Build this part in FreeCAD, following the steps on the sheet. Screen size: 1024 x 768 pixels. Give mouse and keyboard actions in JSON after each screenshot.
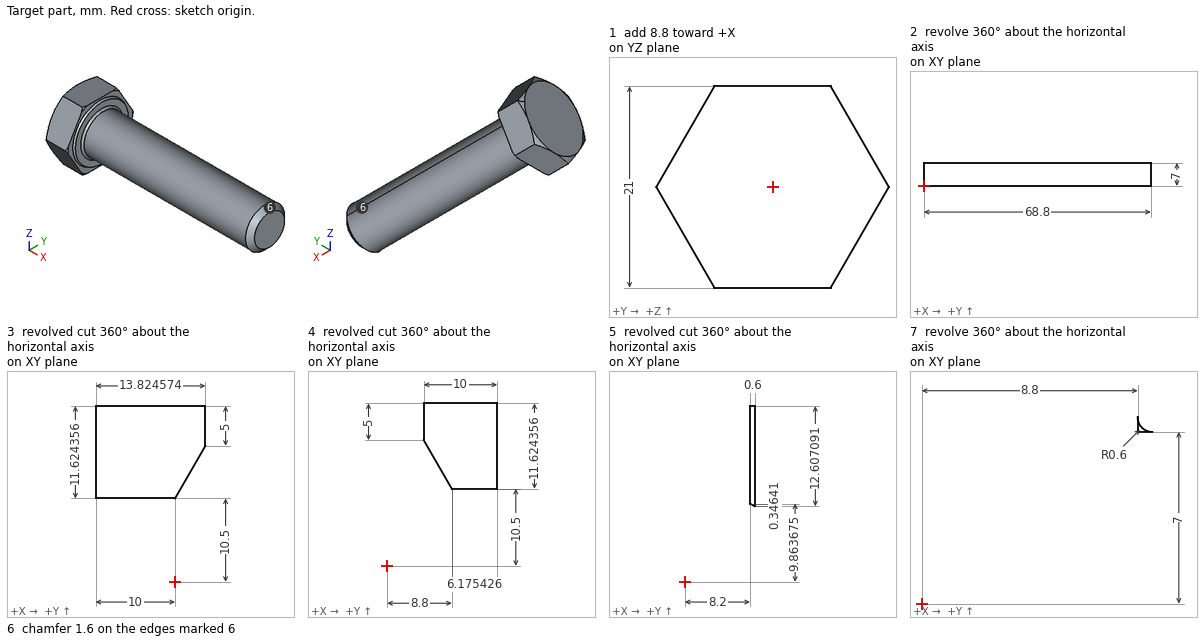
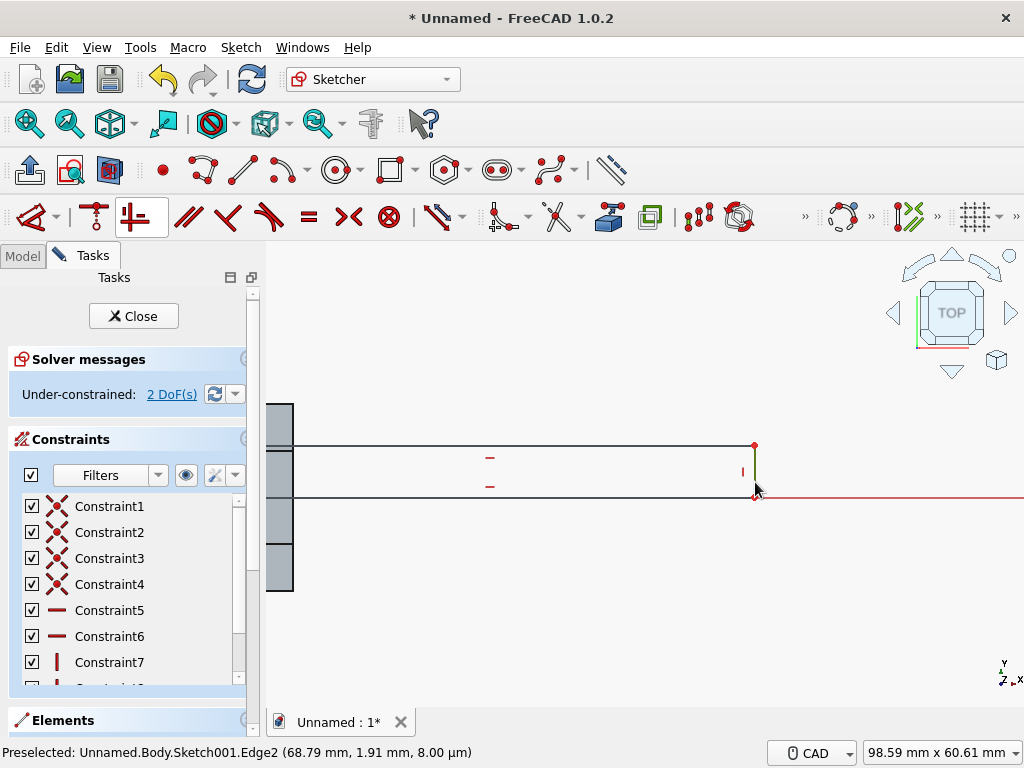
{"action": "left_click", "coordinate": [58, 218]}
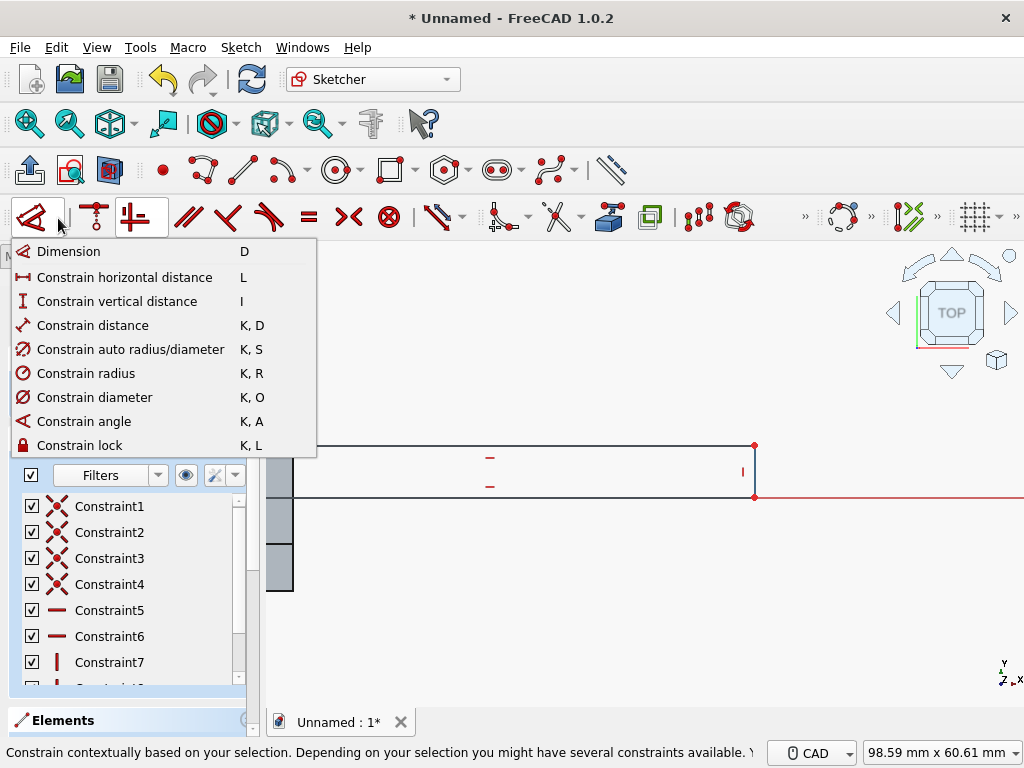
{"action": "left_click", "coordinate": [164, 301]}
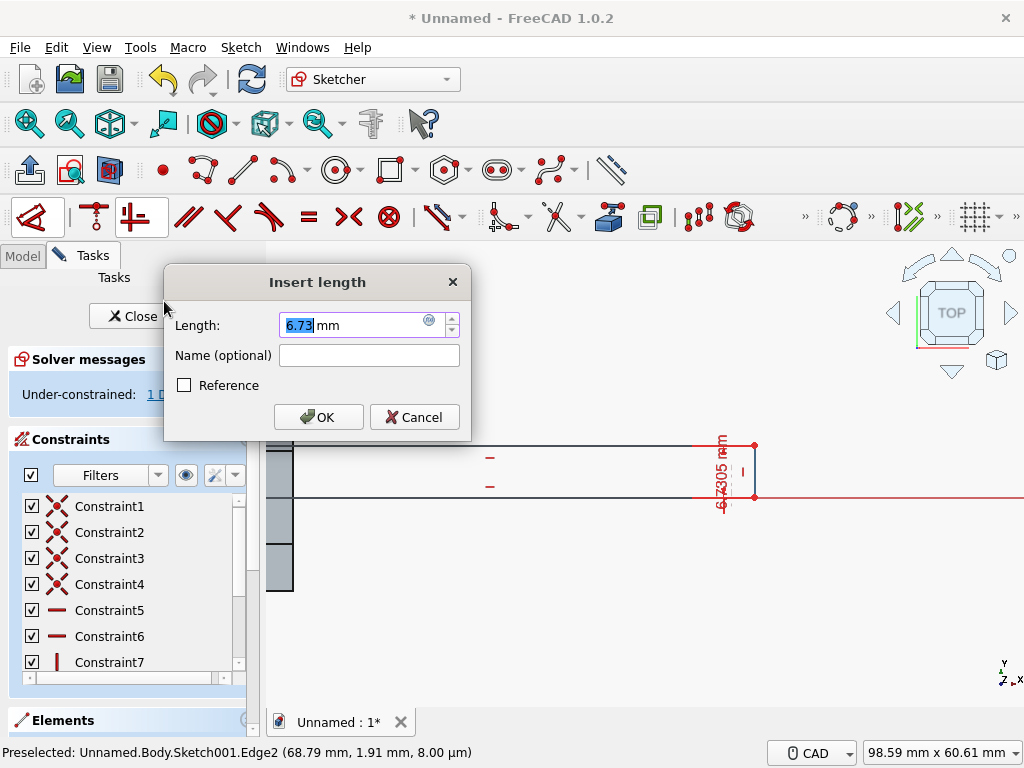
{"action": "type", "text": "7"}
{"action": "key", "text": "Return"}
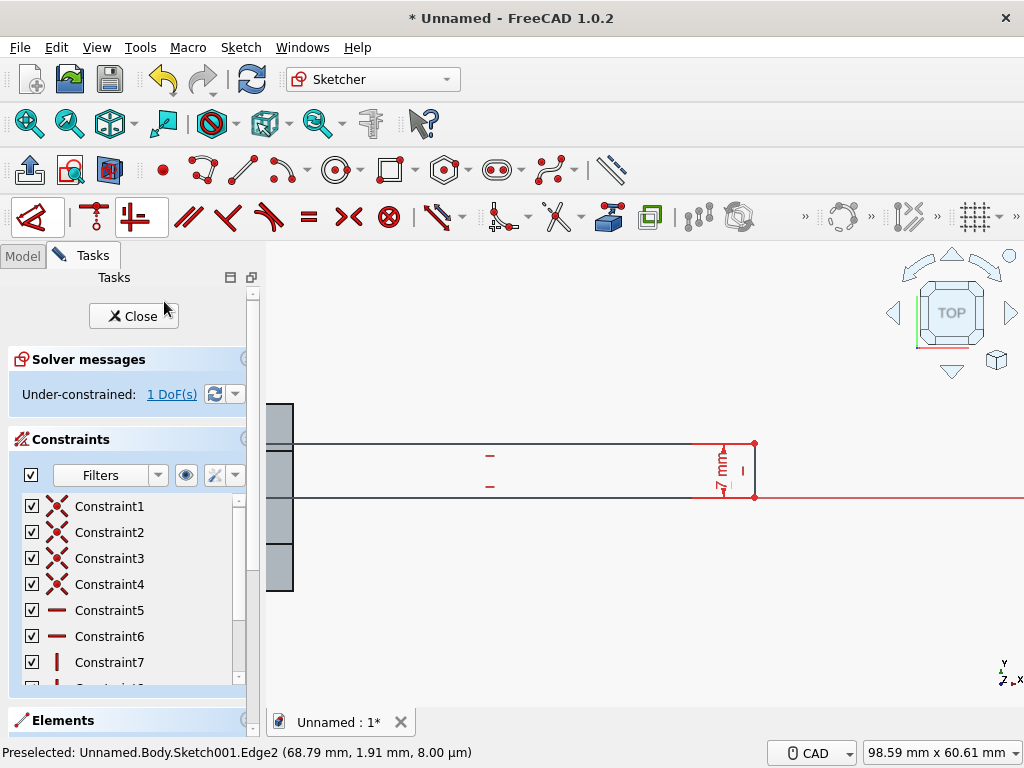
{"action": "left_click", "coordinate": [384, 498]}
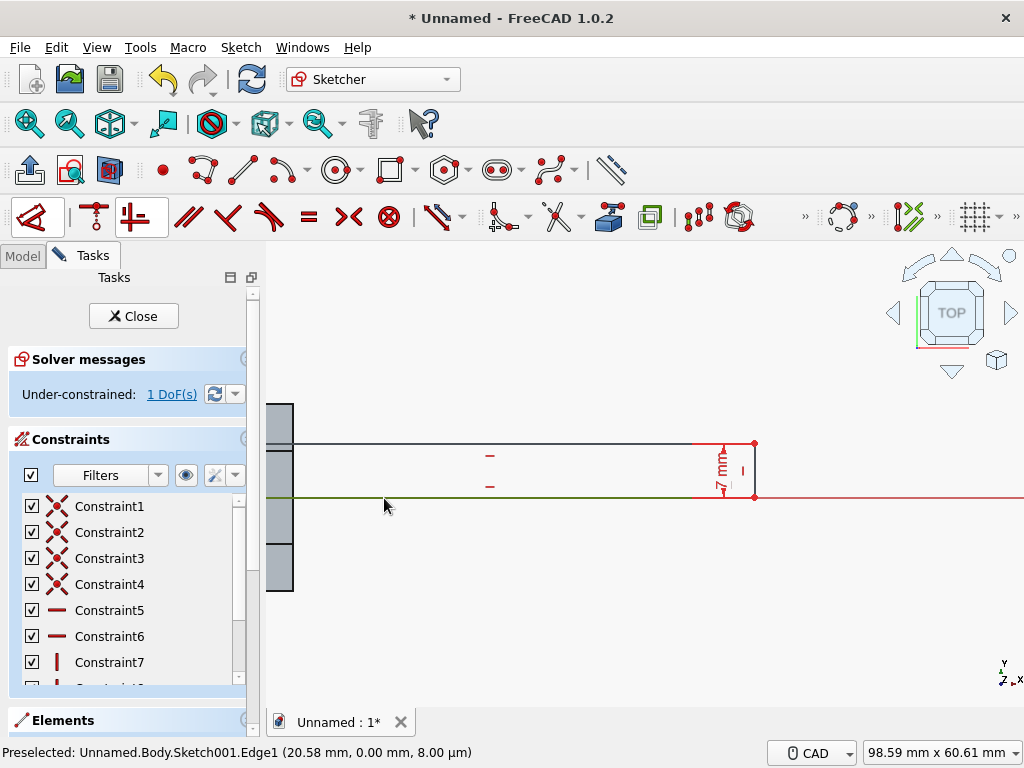
{"action": "left_click", "coordinate": [58, 218]}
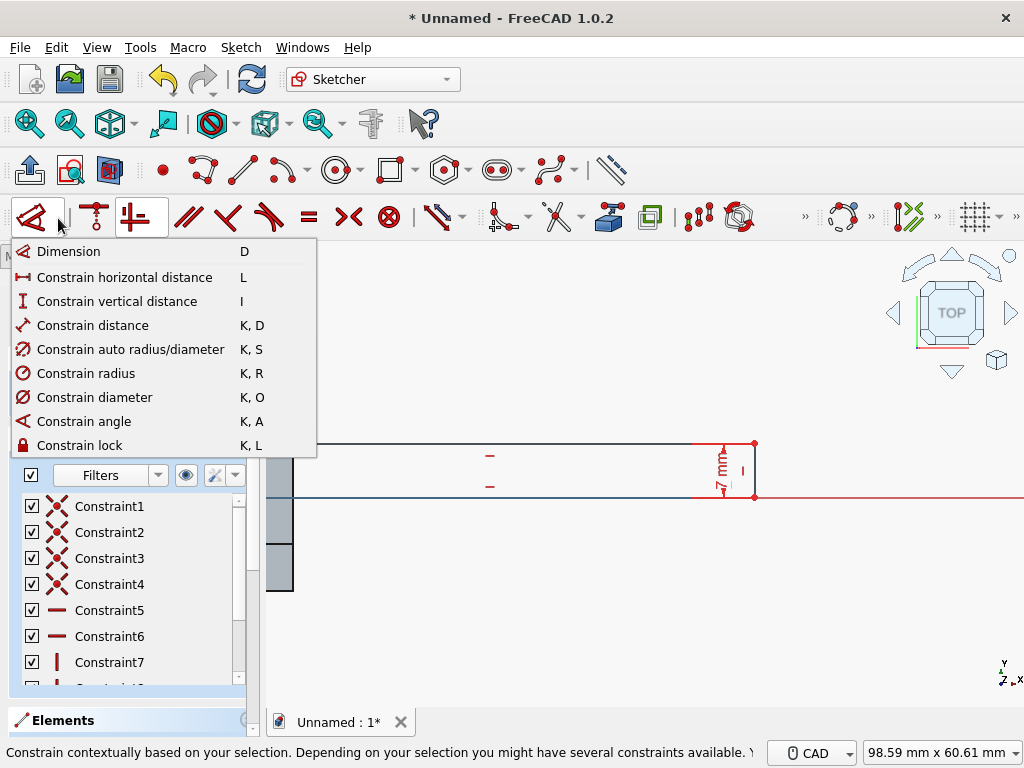
{"action": "left_click", "coordinate": [164, 277]}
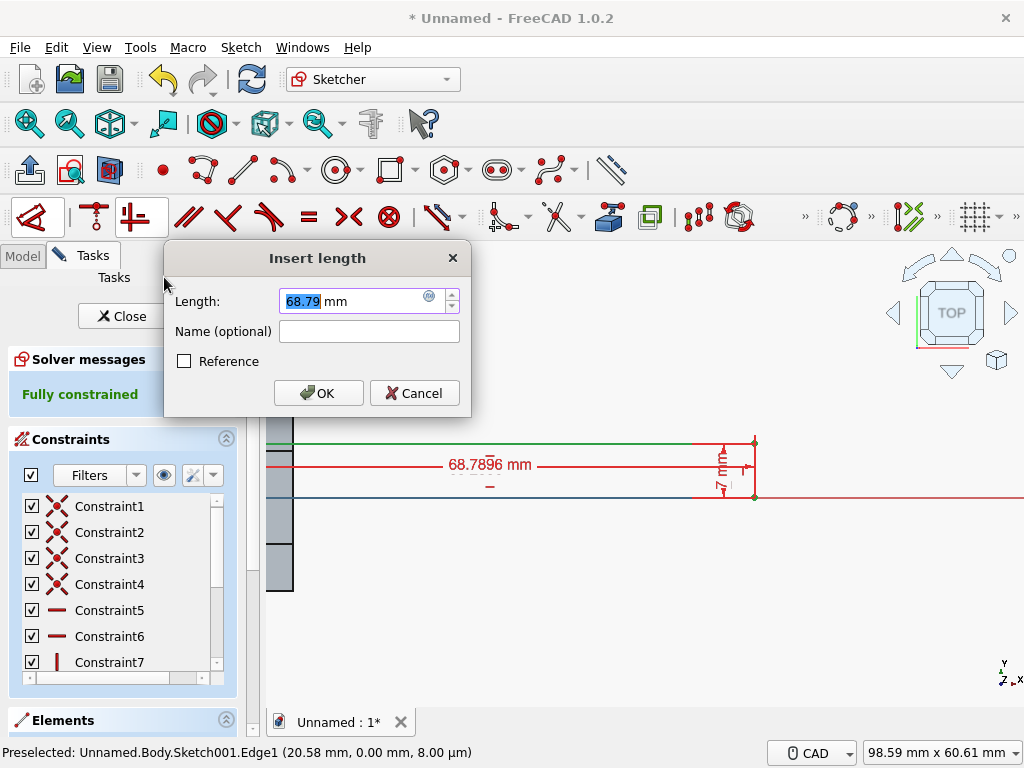
{"action": "type", "text": "68.8"}
{"action": "key", "text": "Return"}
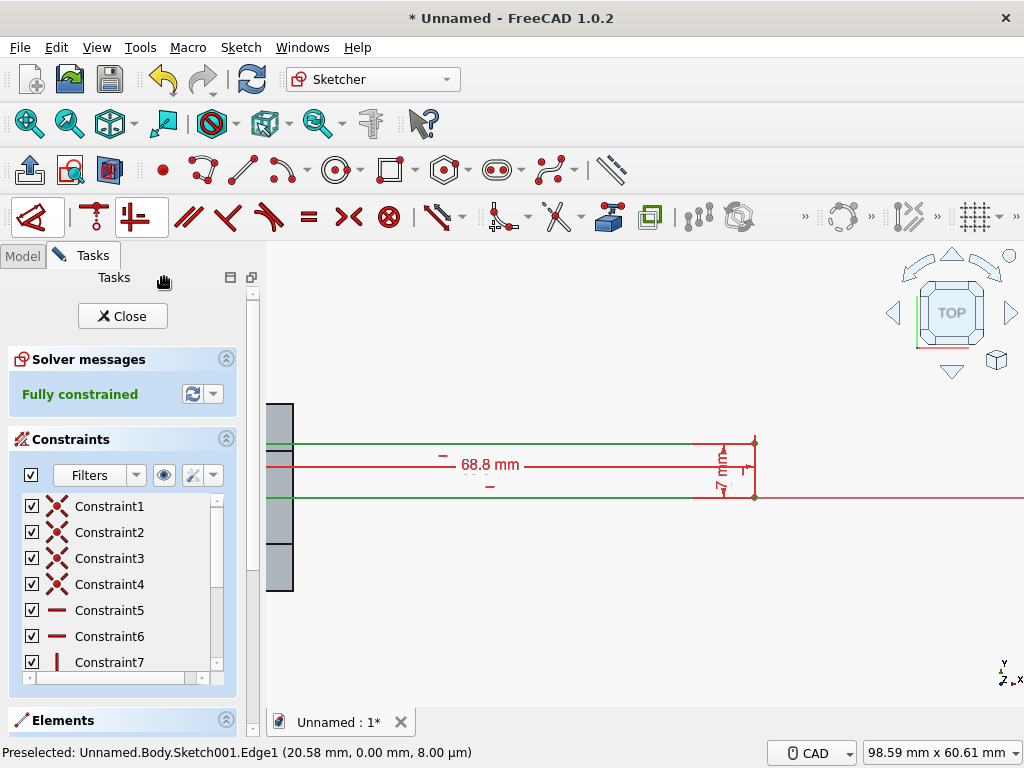
{"action": "left_click", "coordinate": [123, 316]}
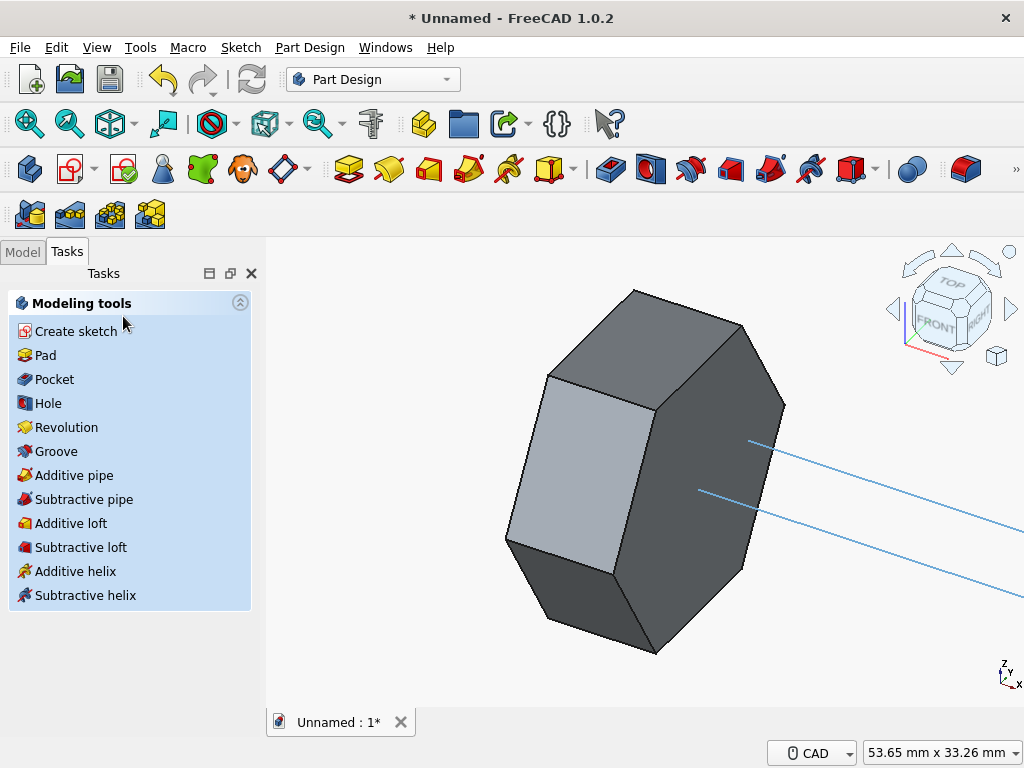
{"action": "left_click", "coordinate": [390, 170]}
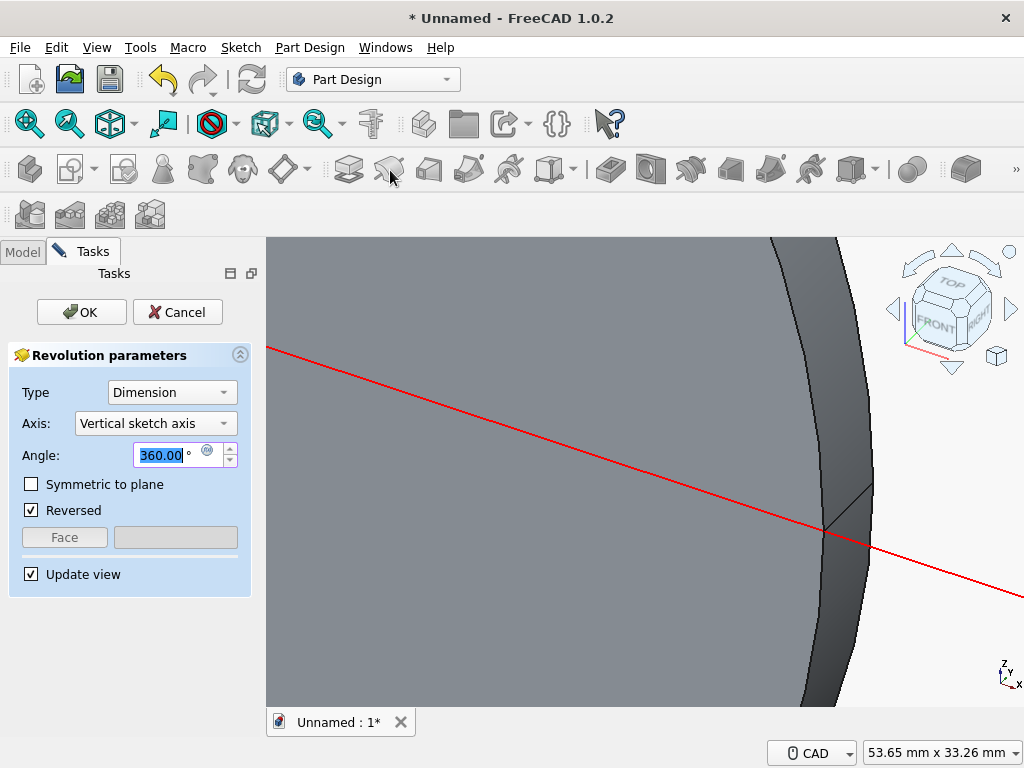
{"action": "left_click", "coordinate": [156, 424]}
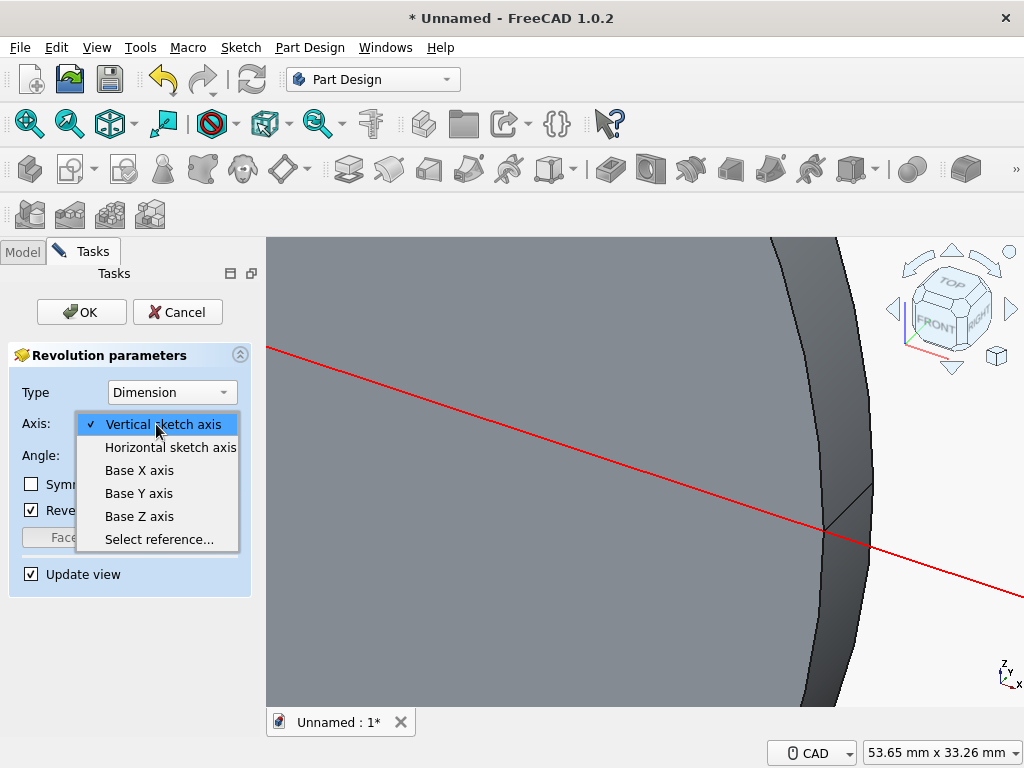
{"action": "left_click", "coordinate": [156, 448]}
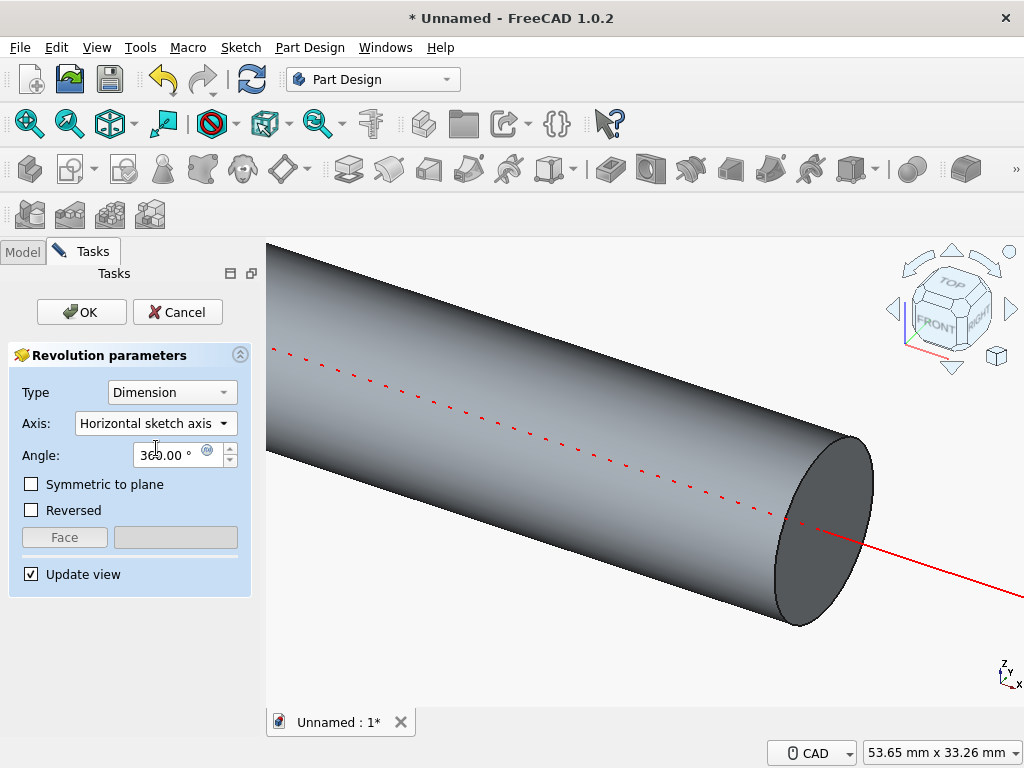
{"action": "left_click", "coordinate": [82, 312]}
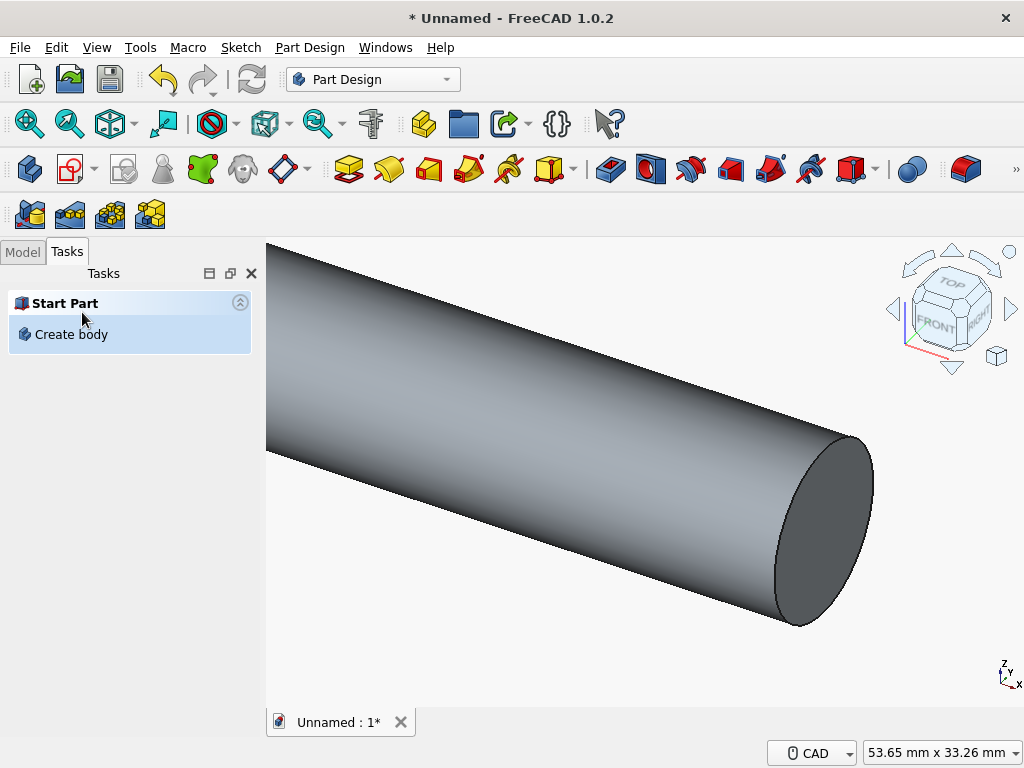
{"action": "left_click", "coordinate": [30, 124]}